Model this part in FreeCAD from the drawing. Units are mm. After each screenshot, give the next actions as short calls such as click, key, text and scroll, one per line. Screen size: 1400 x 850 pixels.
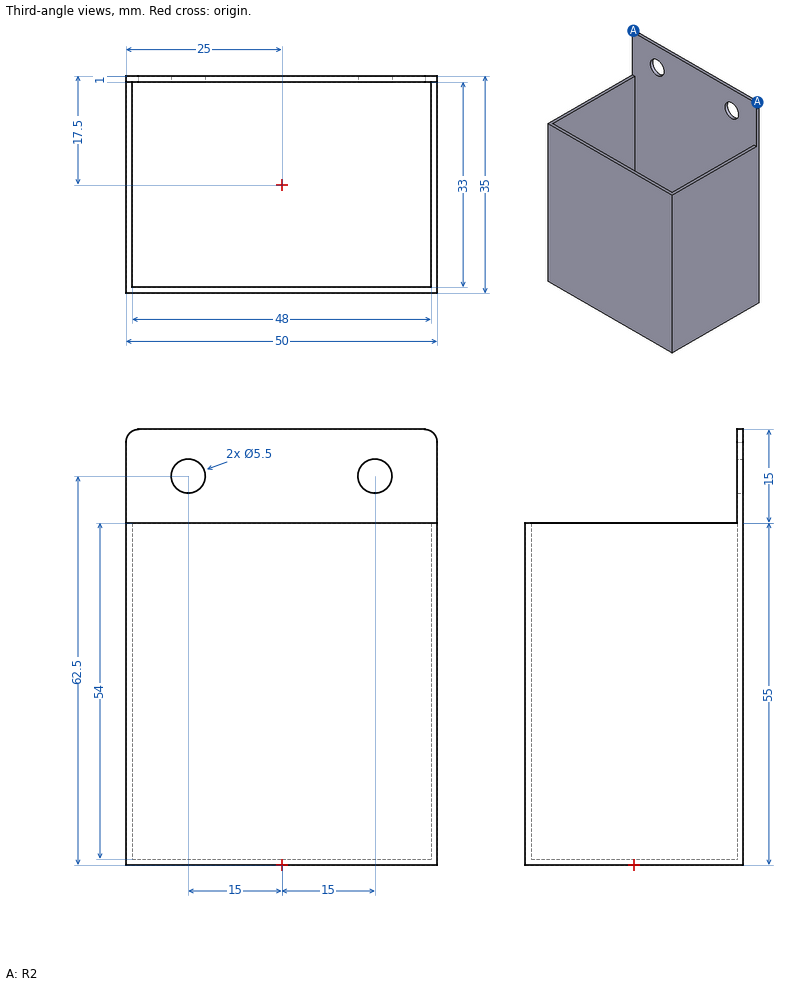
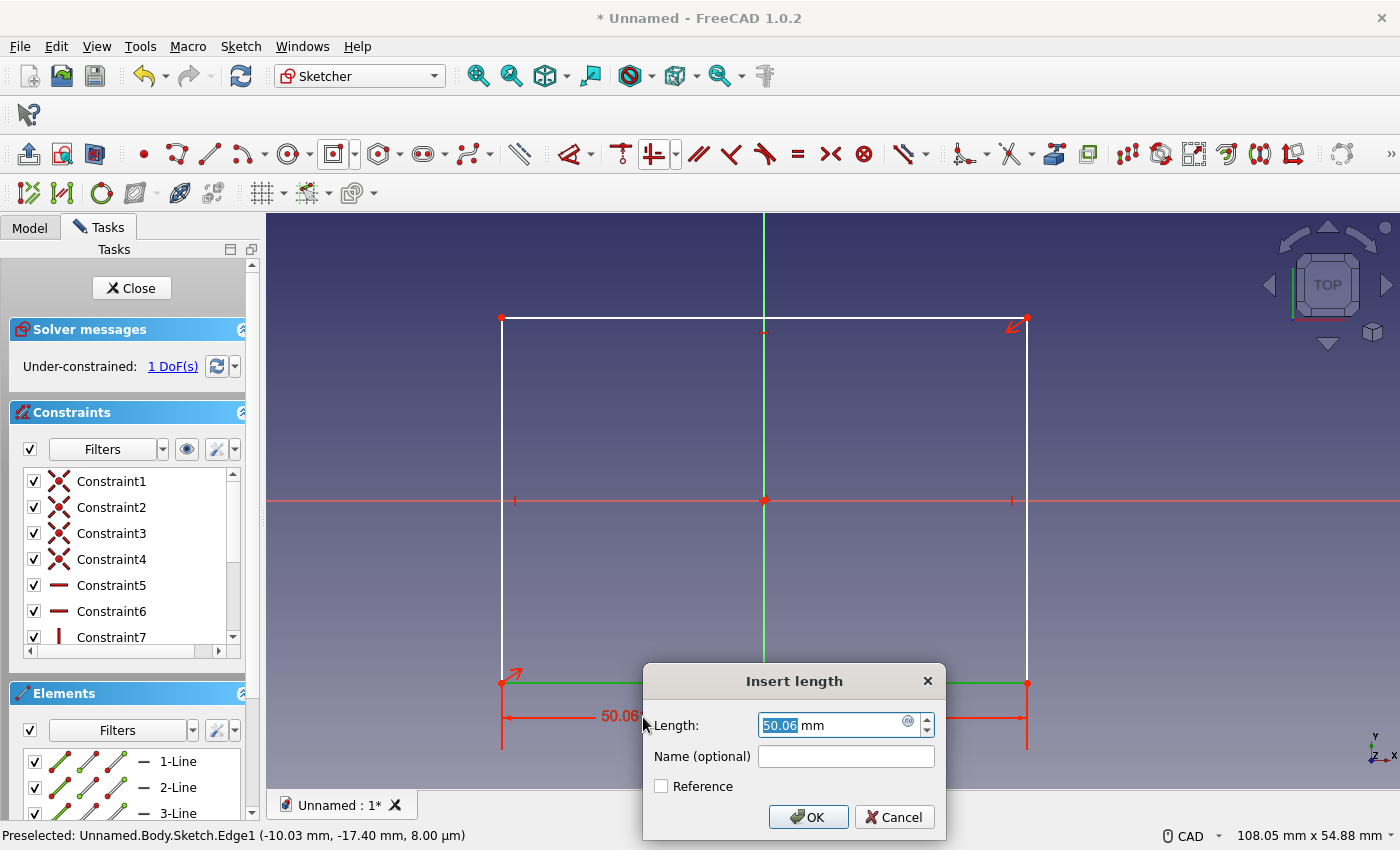
text(50)
key(Return)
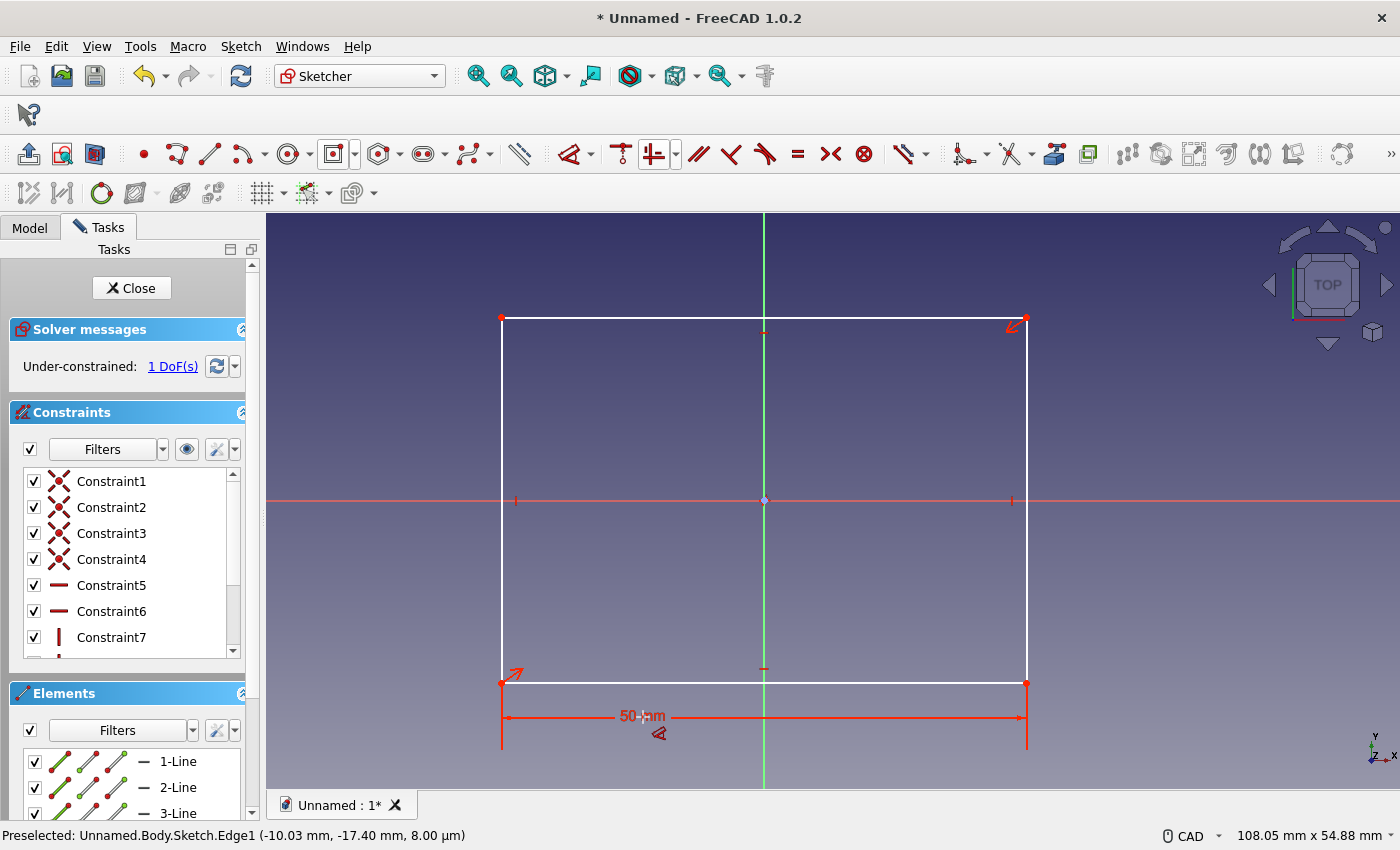
click(1027, 574)
click(1061, 417)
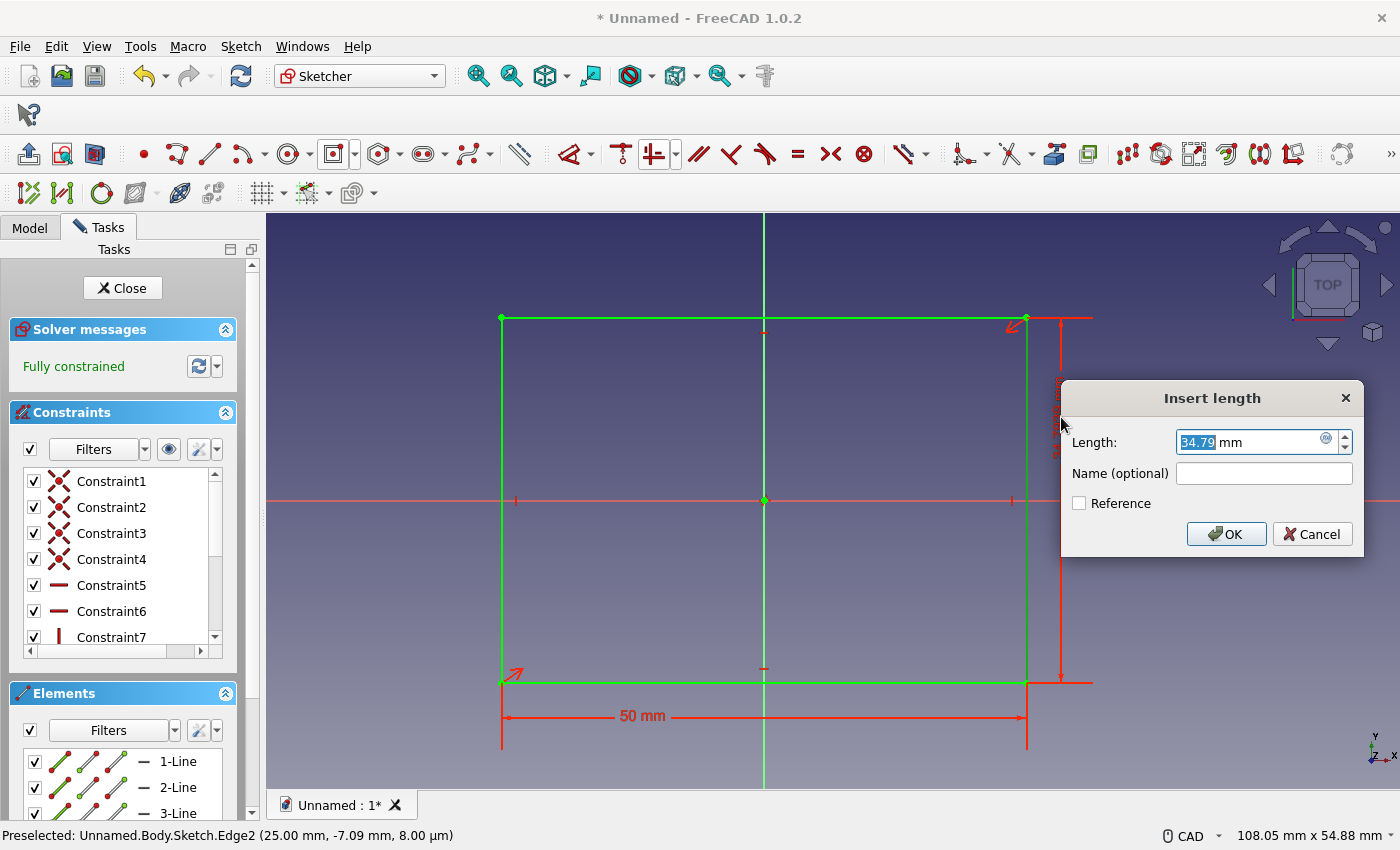
text(35)
key(Return)
key(Escape)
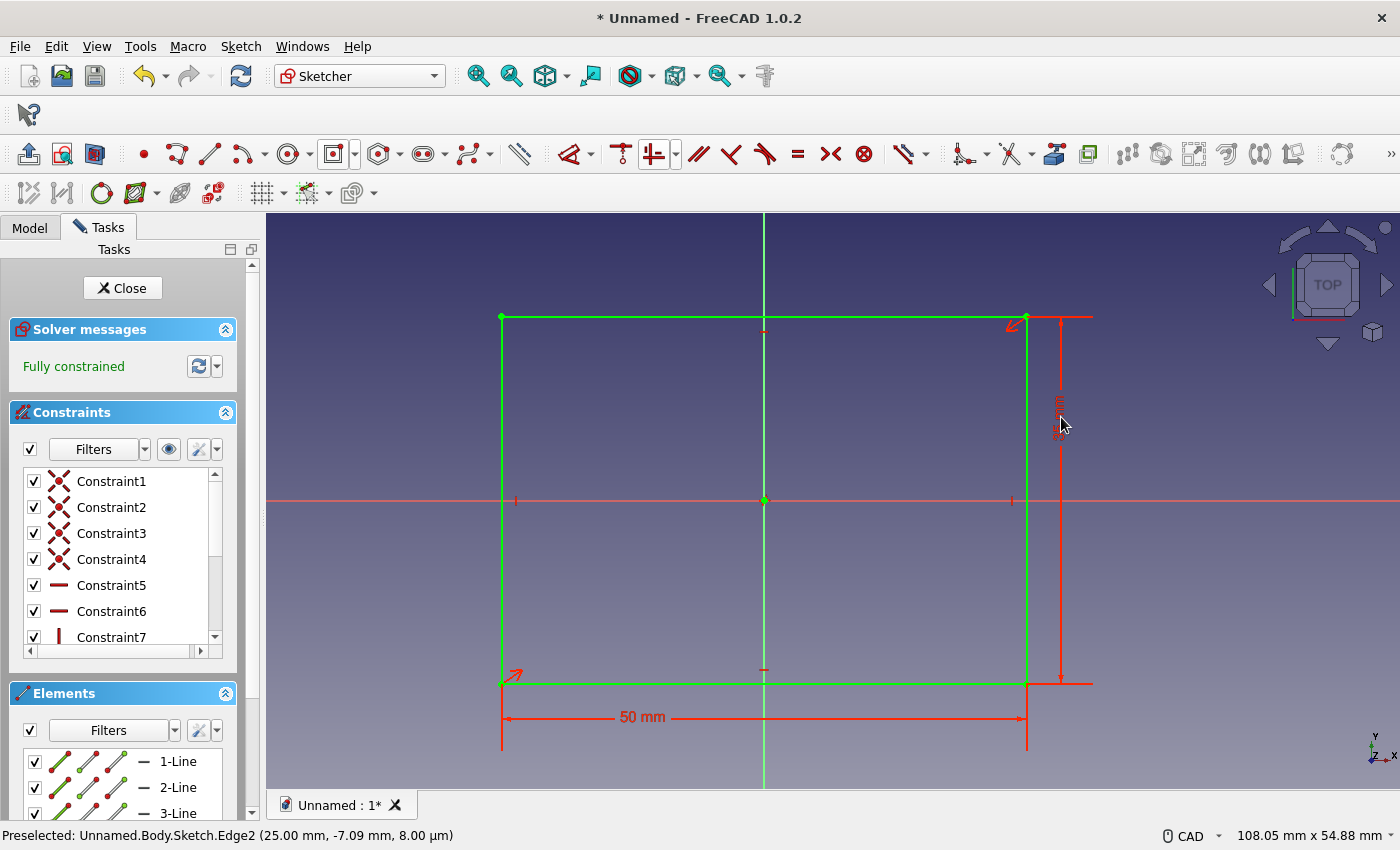
click(123, 288)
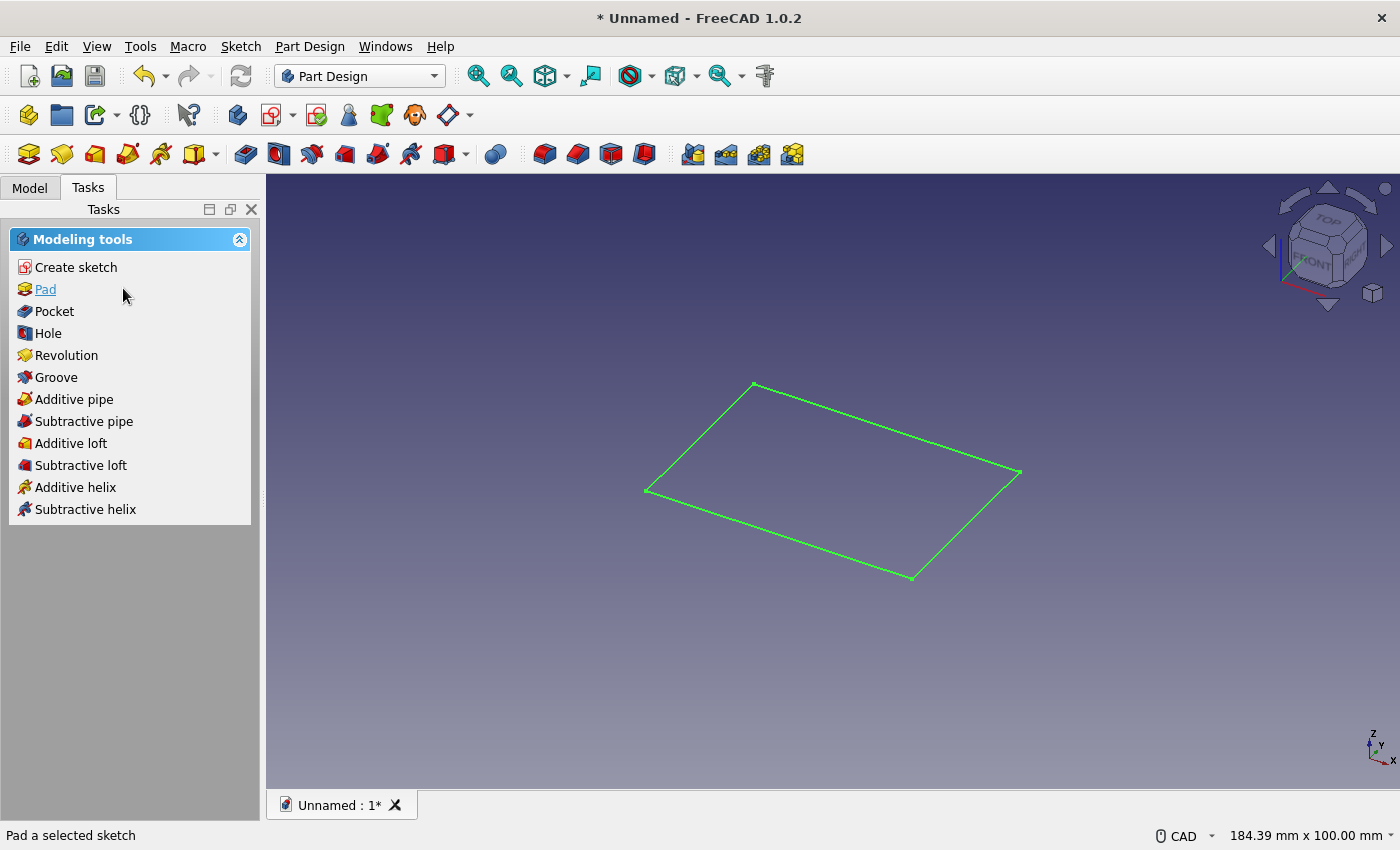
click(29, 154)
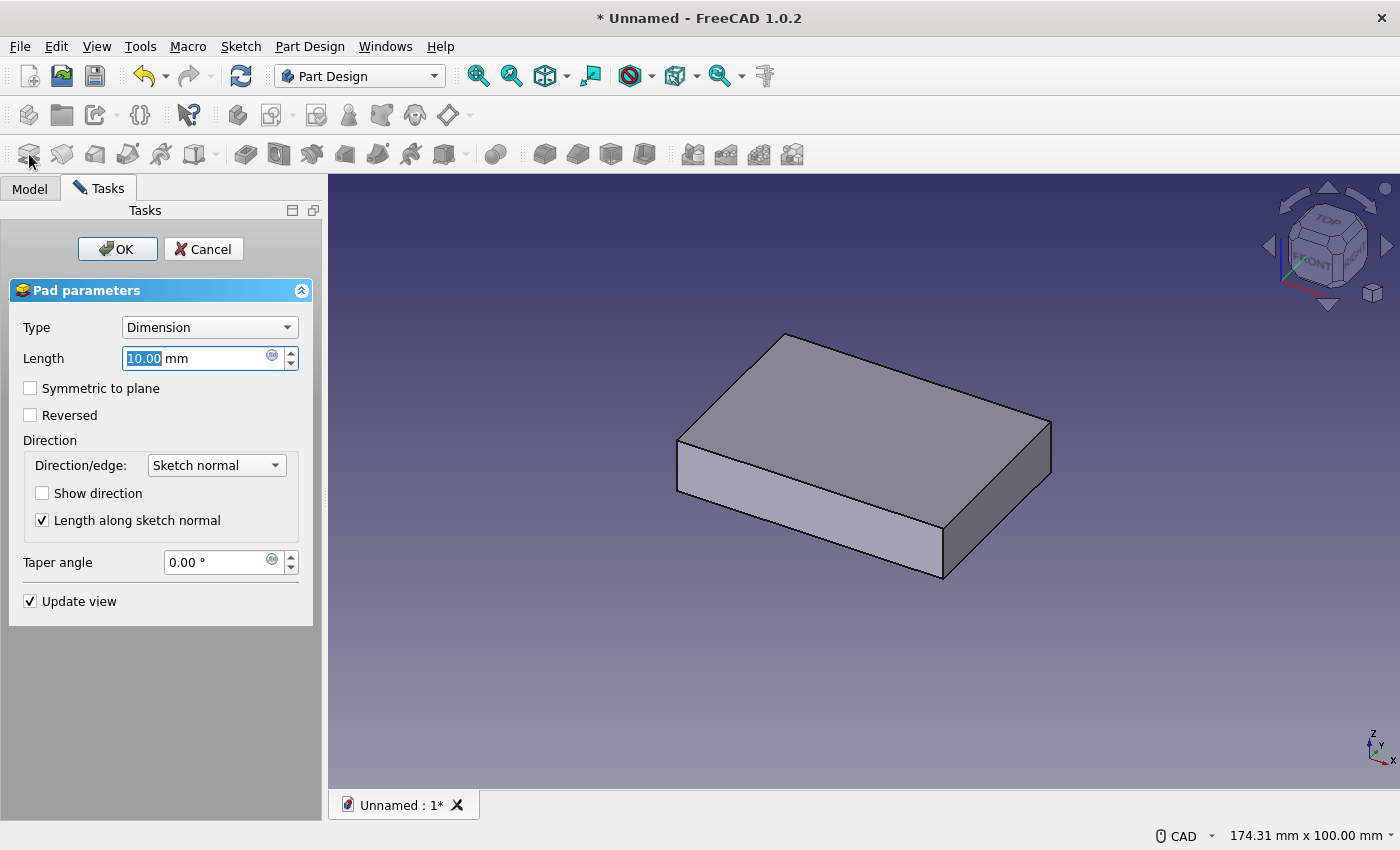
text(55)
key(Tab)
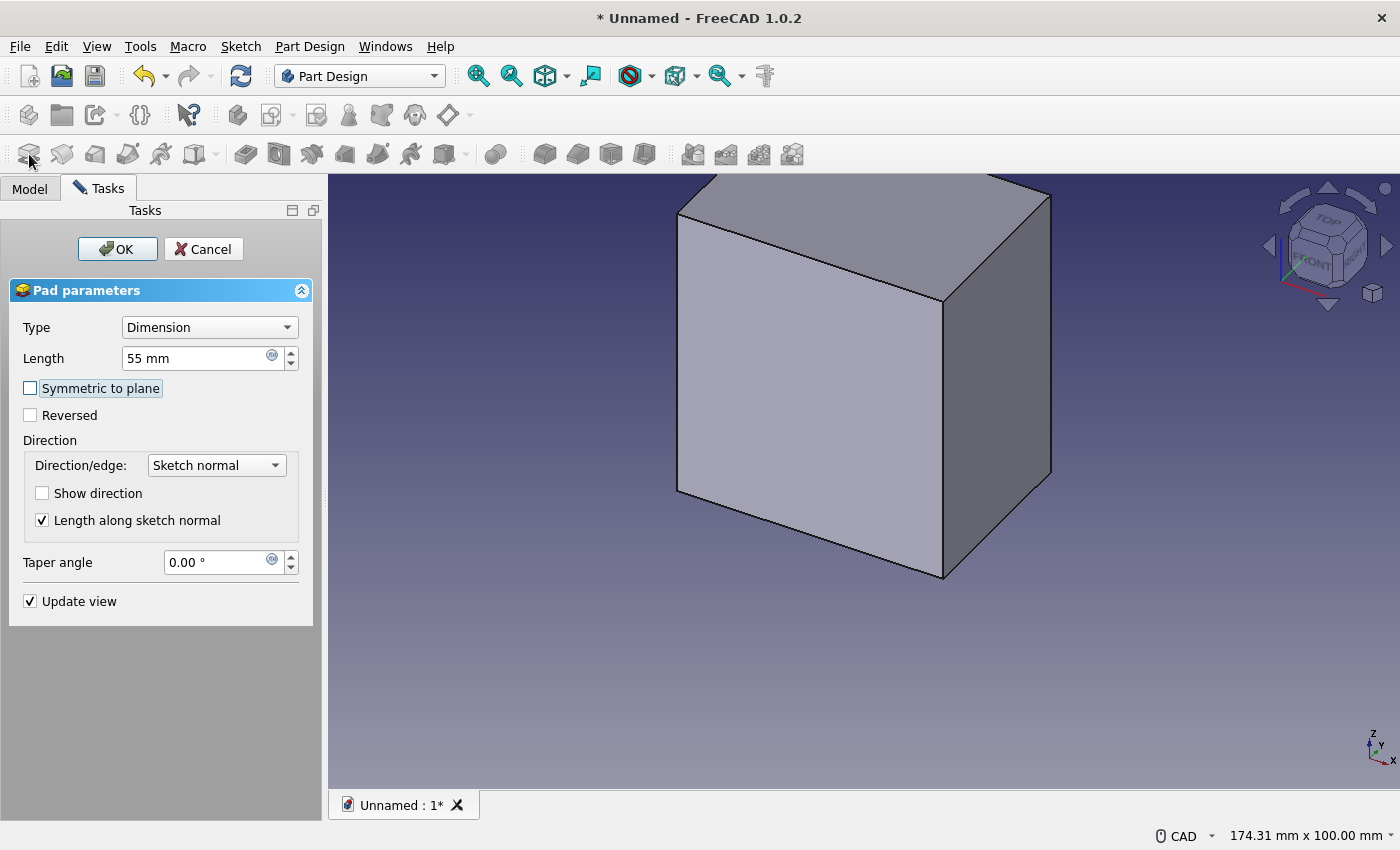
click(118, 249)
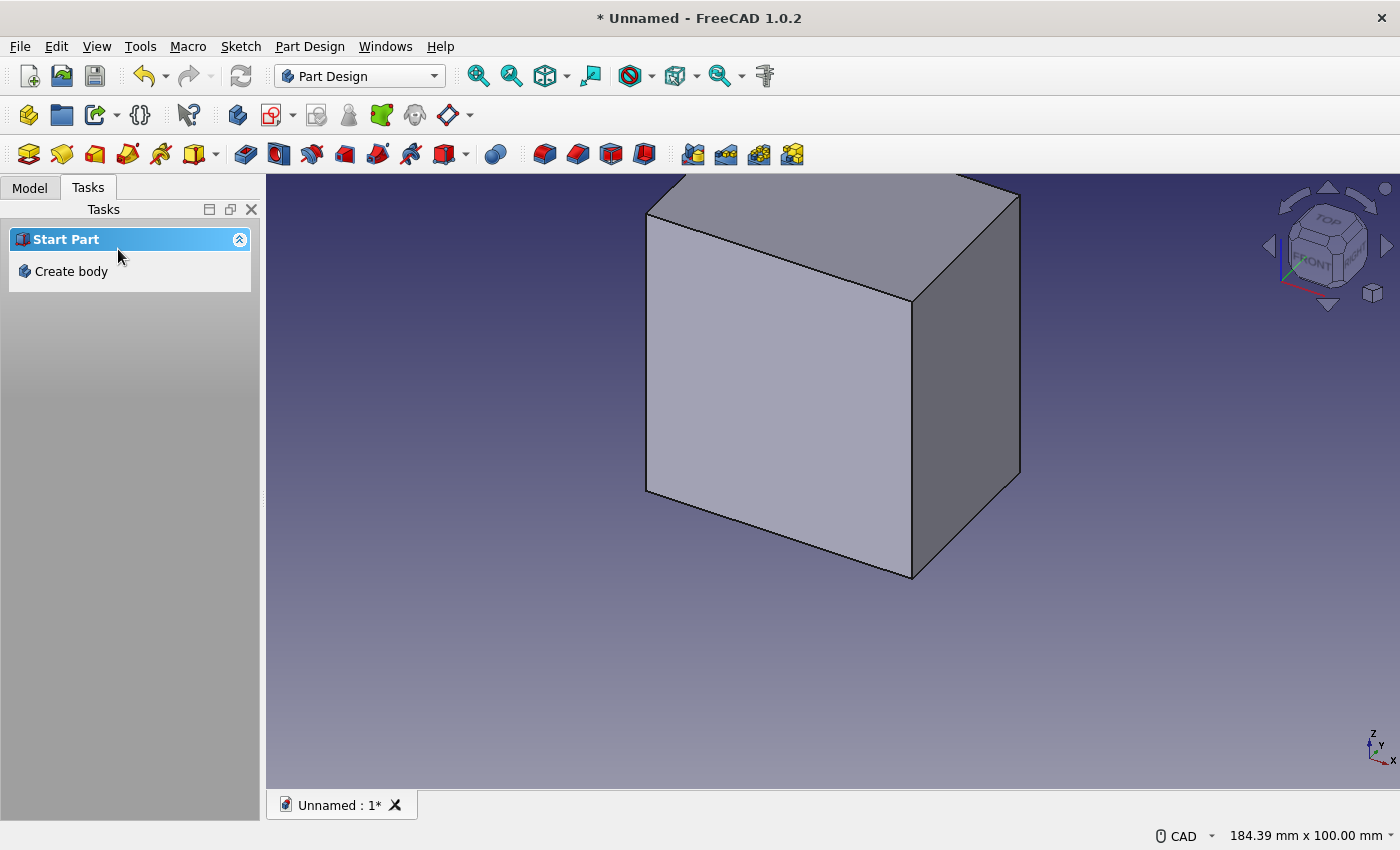
click(479, 76)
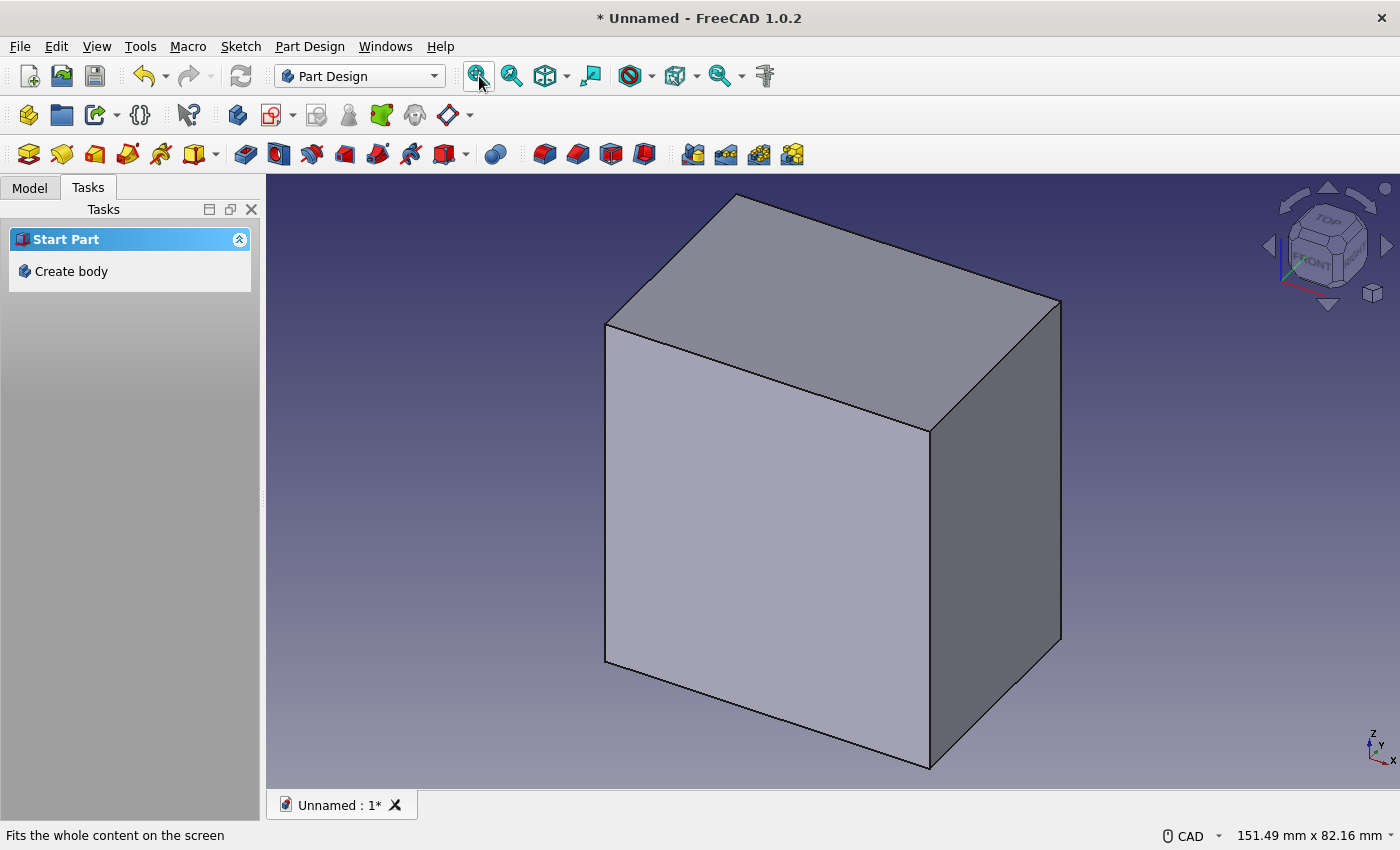
click(879, 327)